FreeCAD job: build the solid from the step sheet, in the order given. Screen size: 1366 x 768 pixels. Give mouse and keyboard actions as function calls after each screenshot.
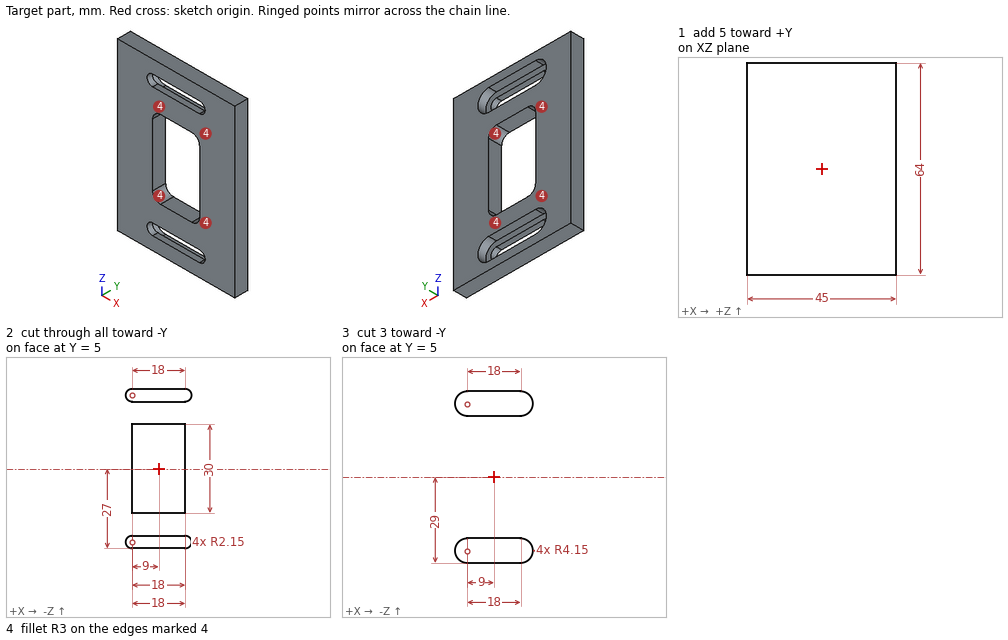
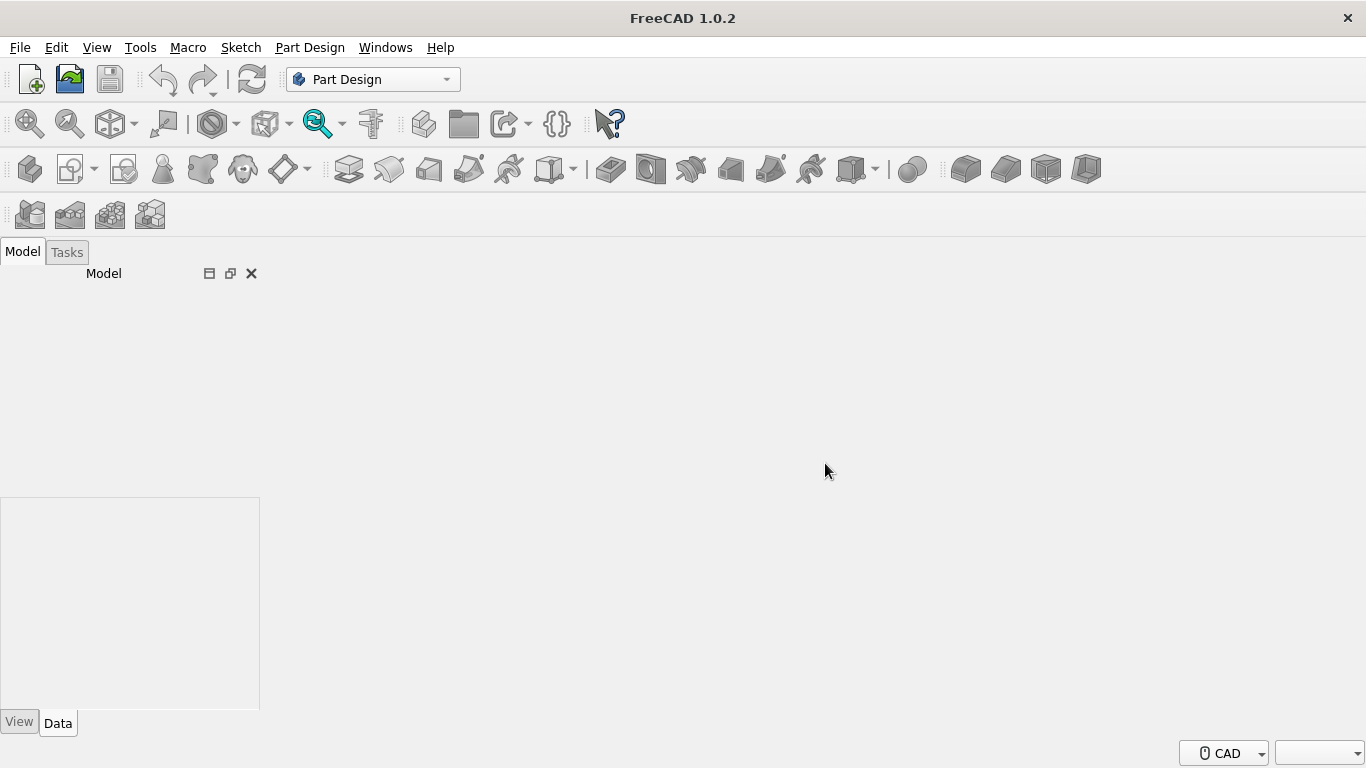
click(30, 80)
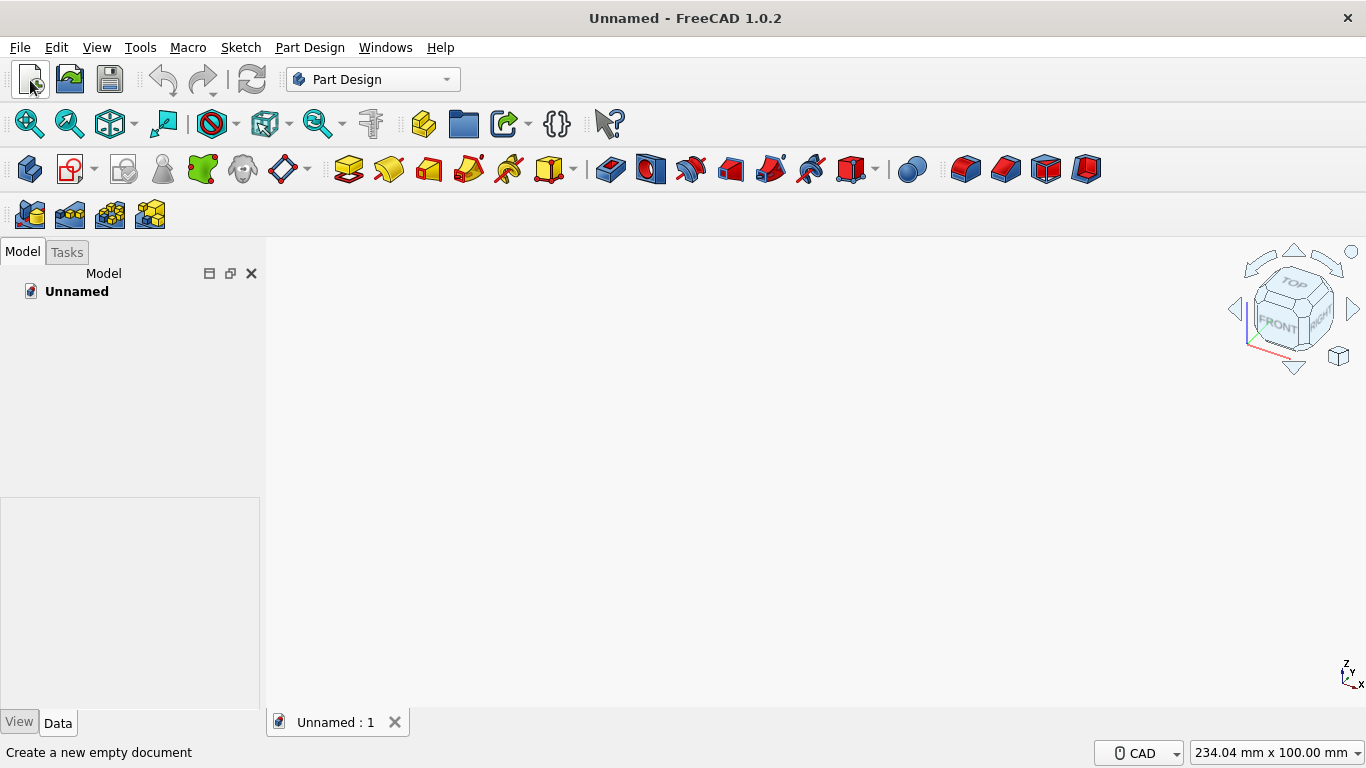
click(70, 170)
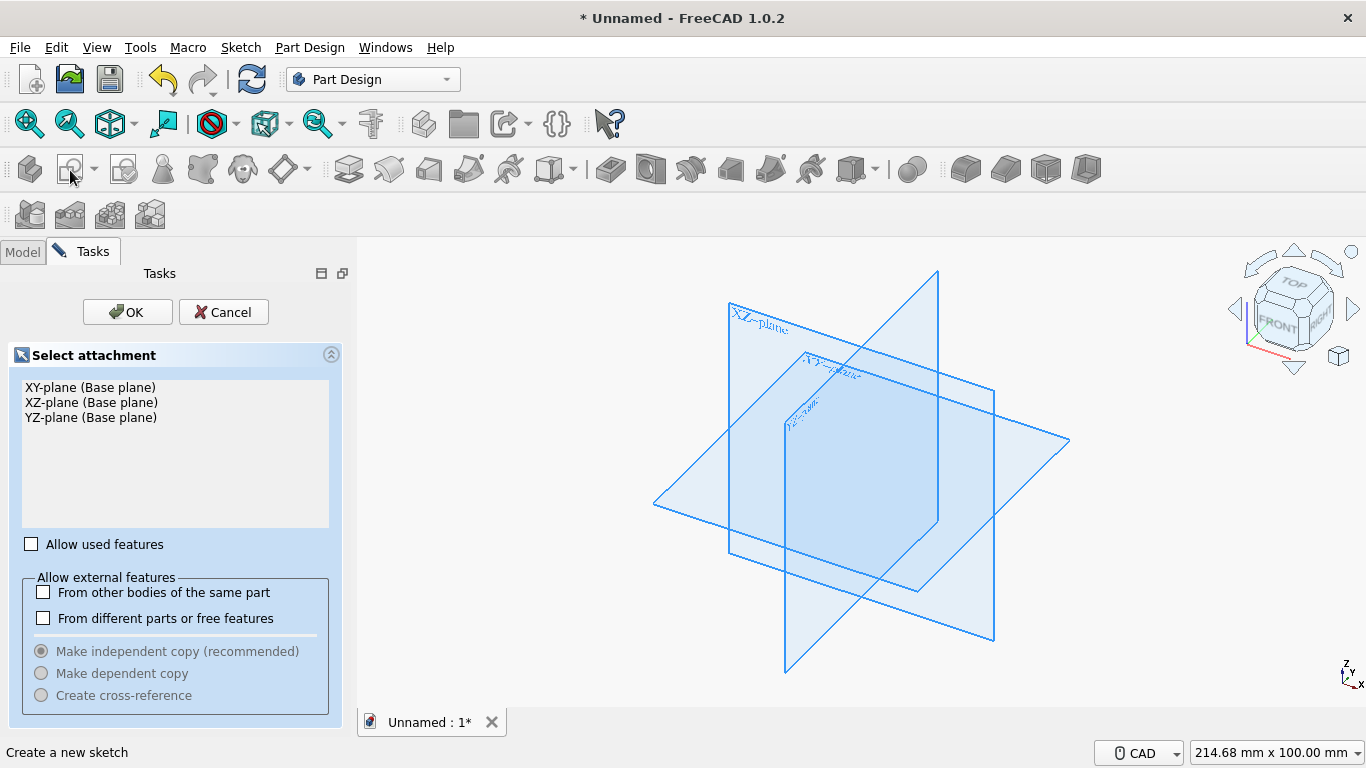
click(82, 402)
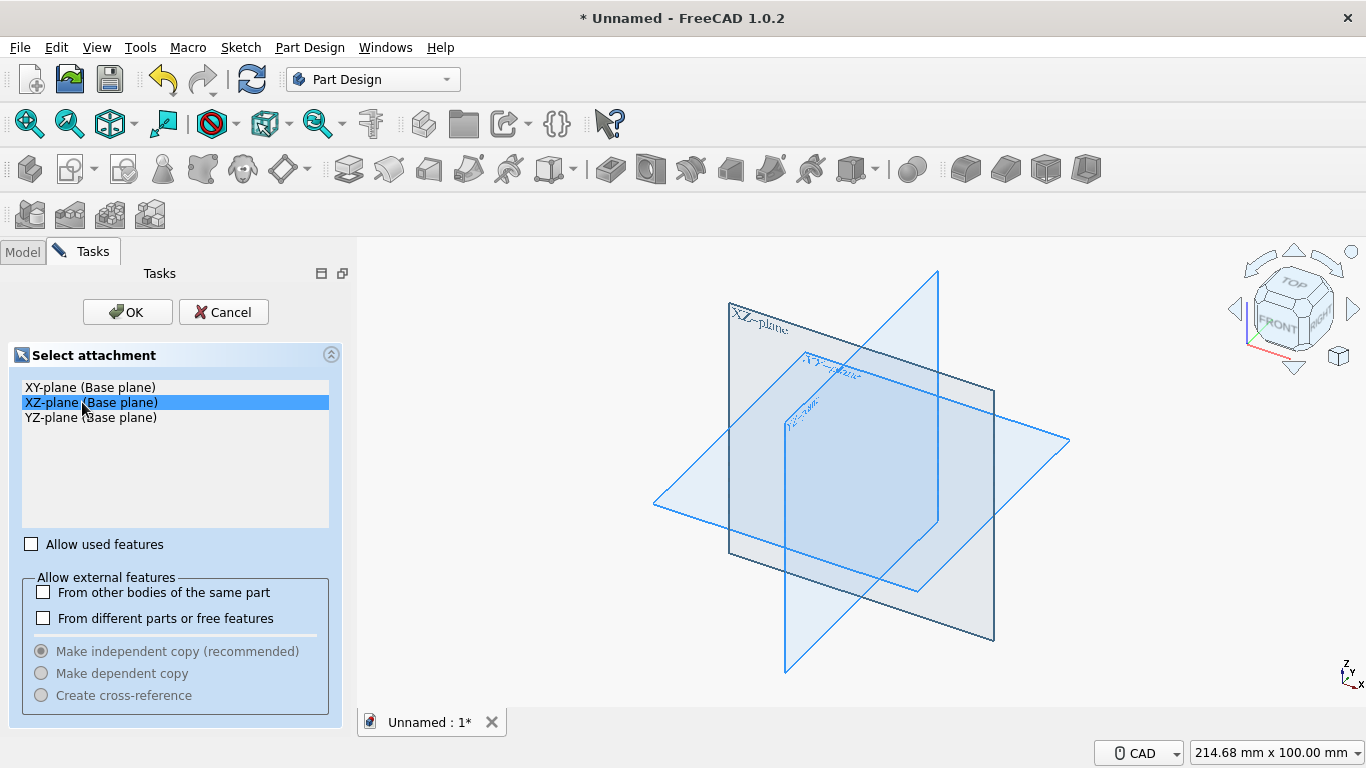
click(128, 312)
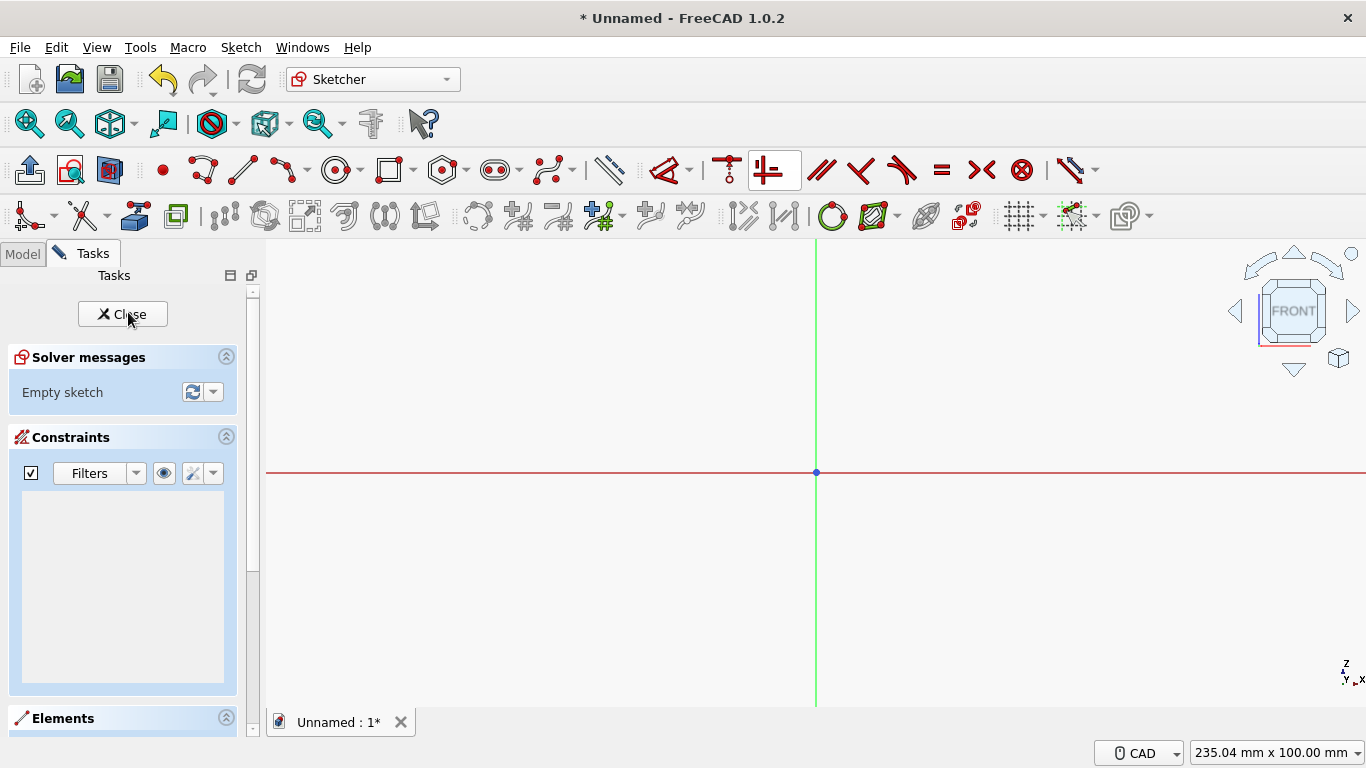
key(g)
key(v)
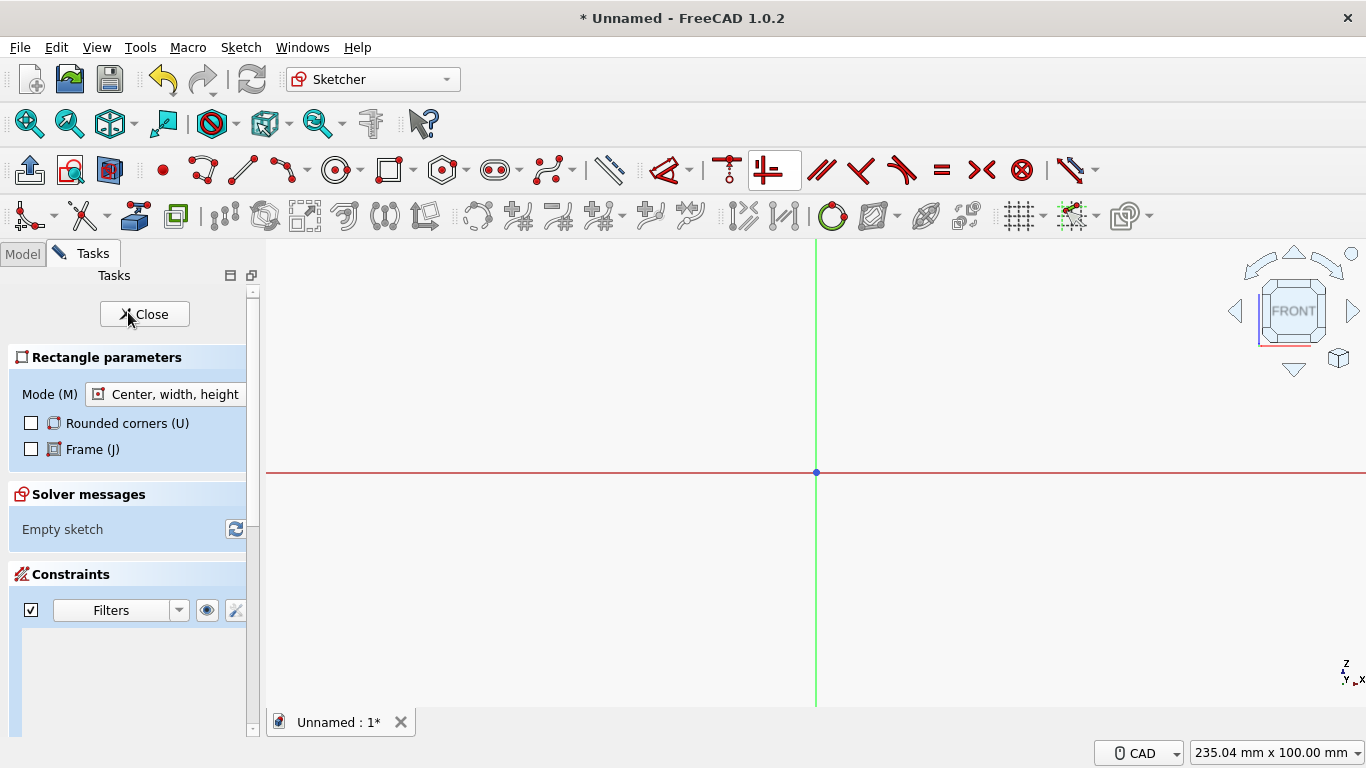
click(816, 473)
click(921, 323)
key(Escape)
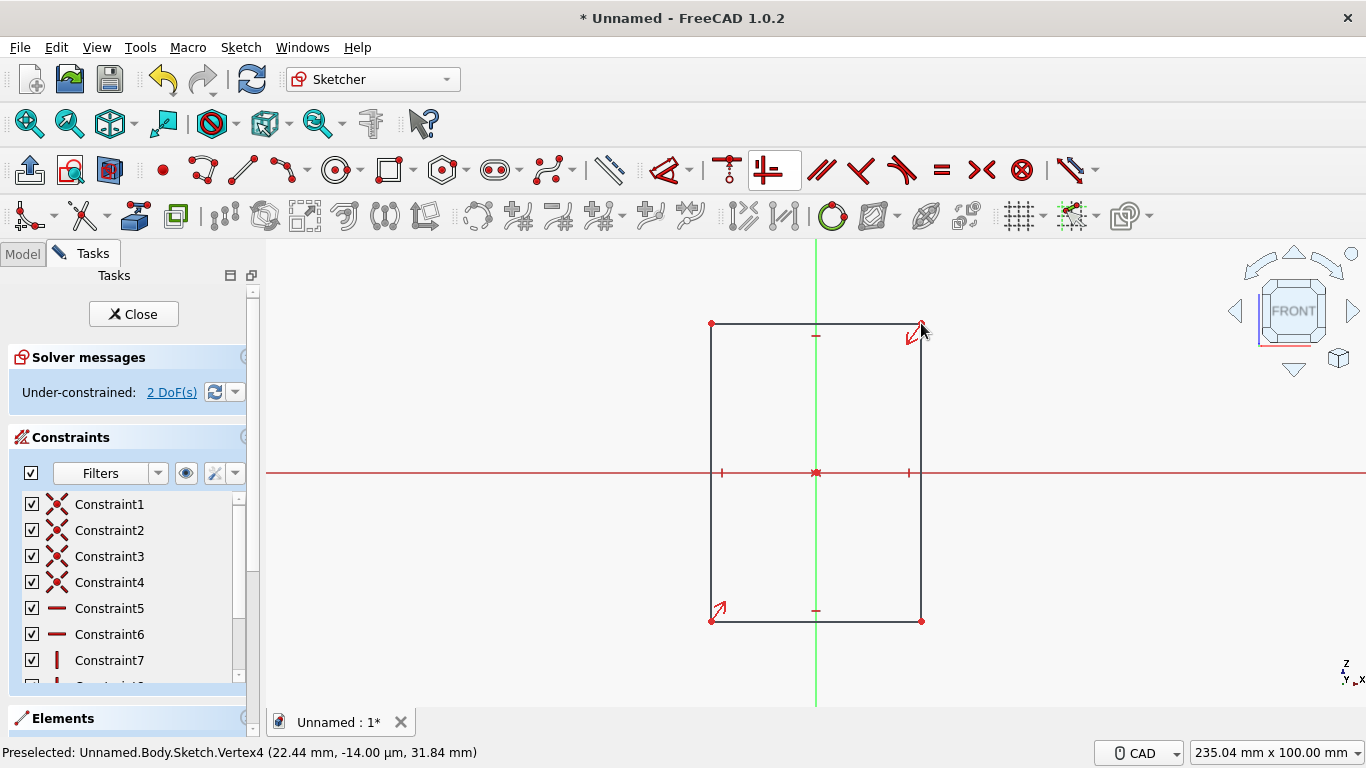
click(664, 170)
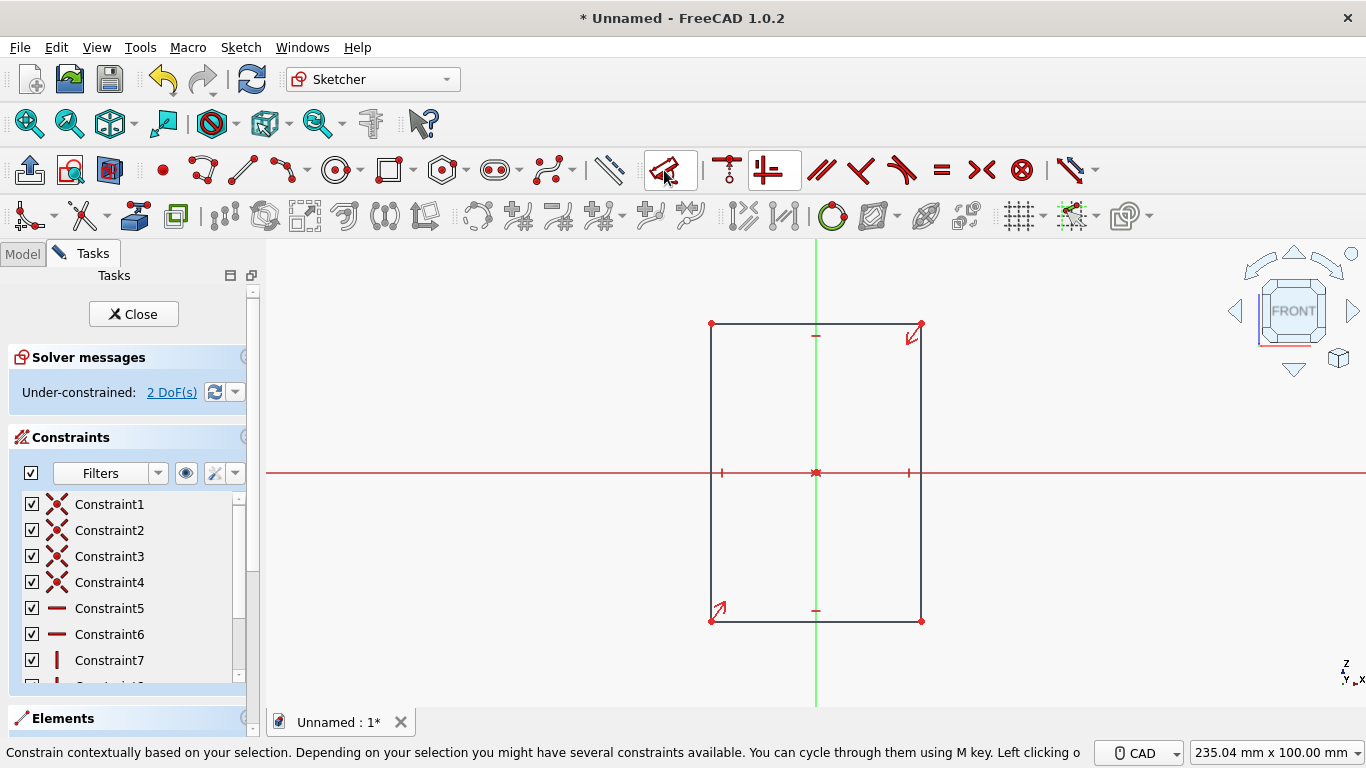
click(774, 622)
click(768, 656)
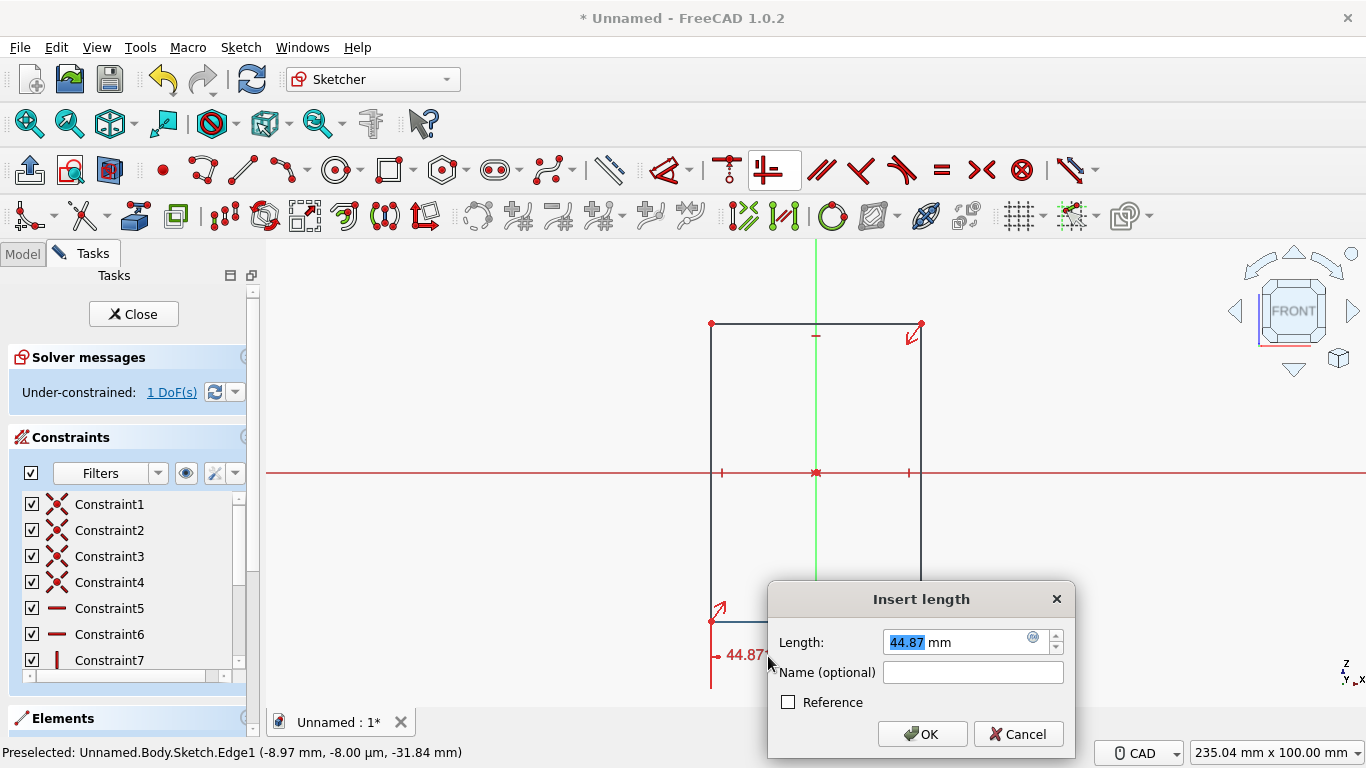
text(45)
key(Return)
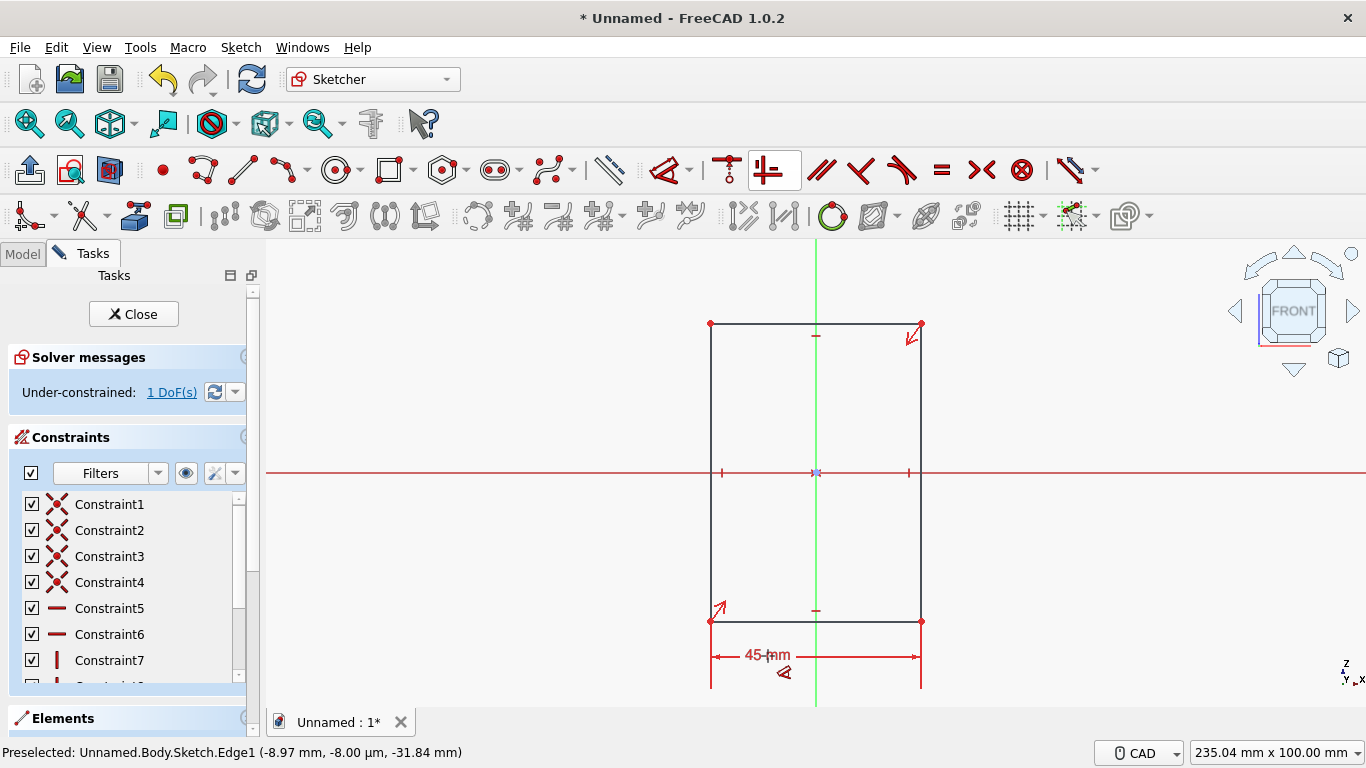
click(921, 533)
click(955, 404)